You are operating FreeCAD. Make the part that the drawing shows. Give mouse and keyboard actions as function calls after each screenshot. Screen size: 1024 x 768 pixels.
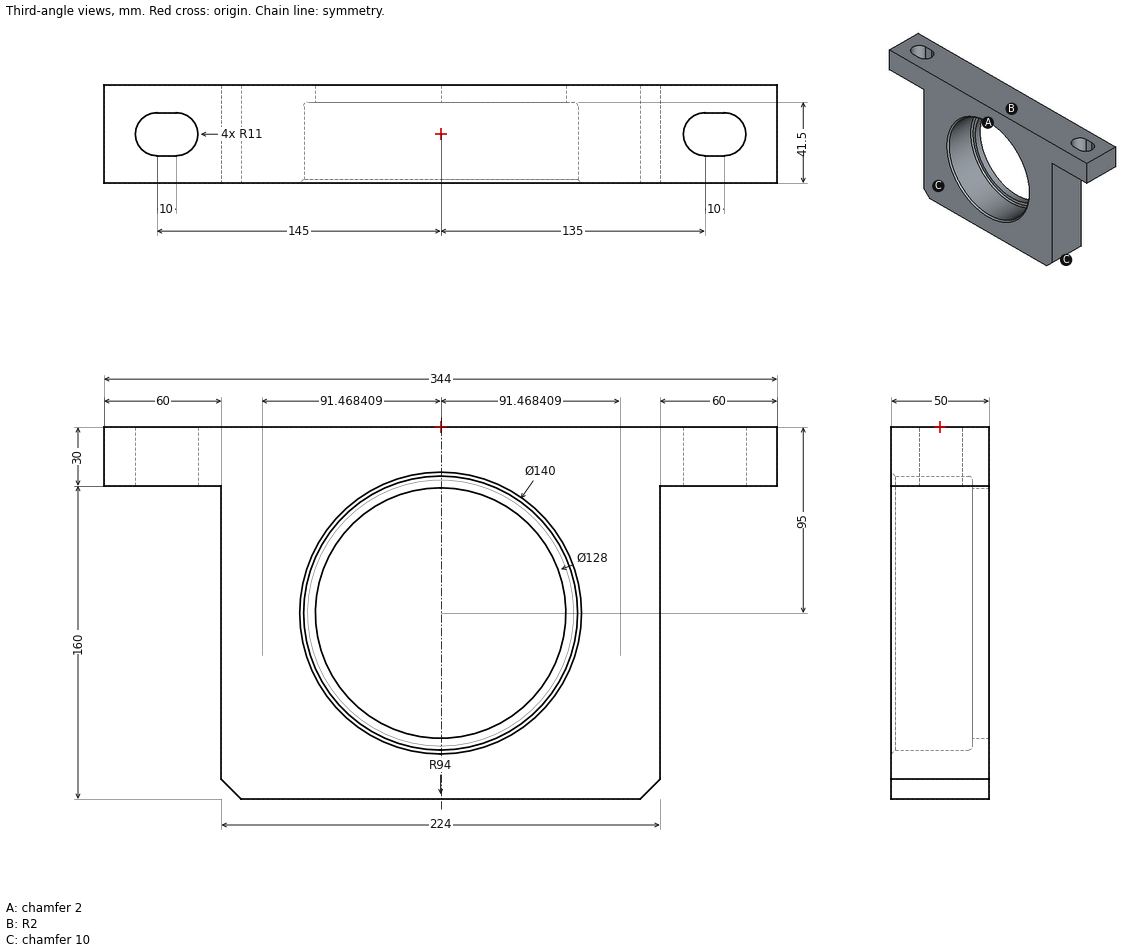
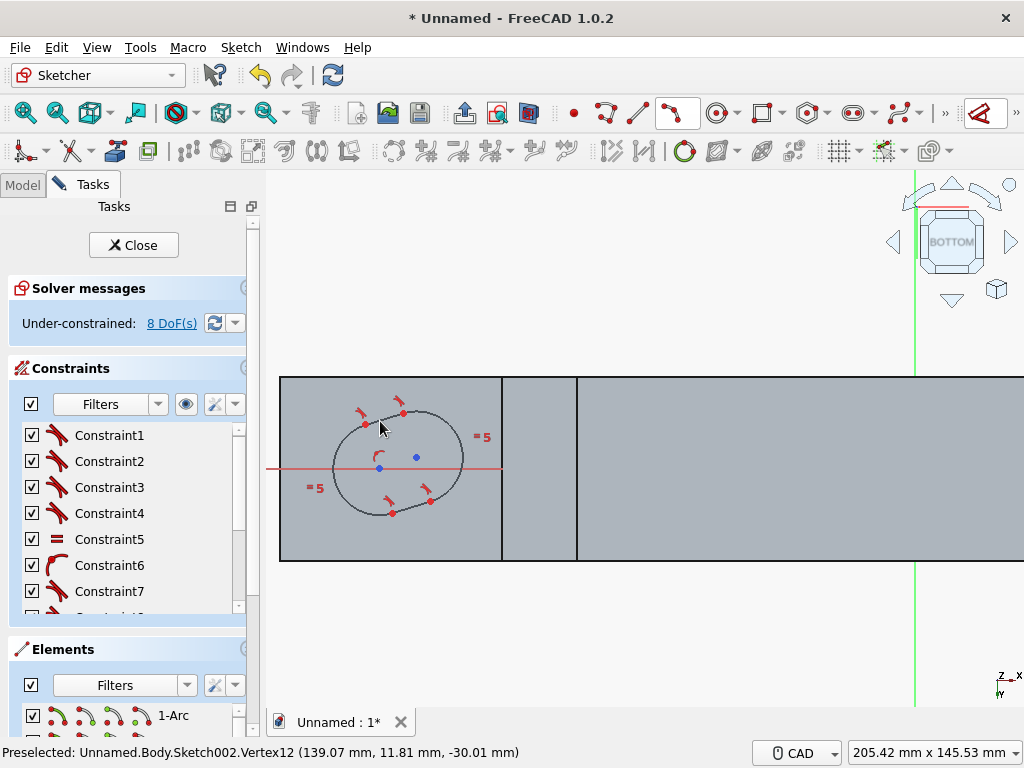
click(381, 420)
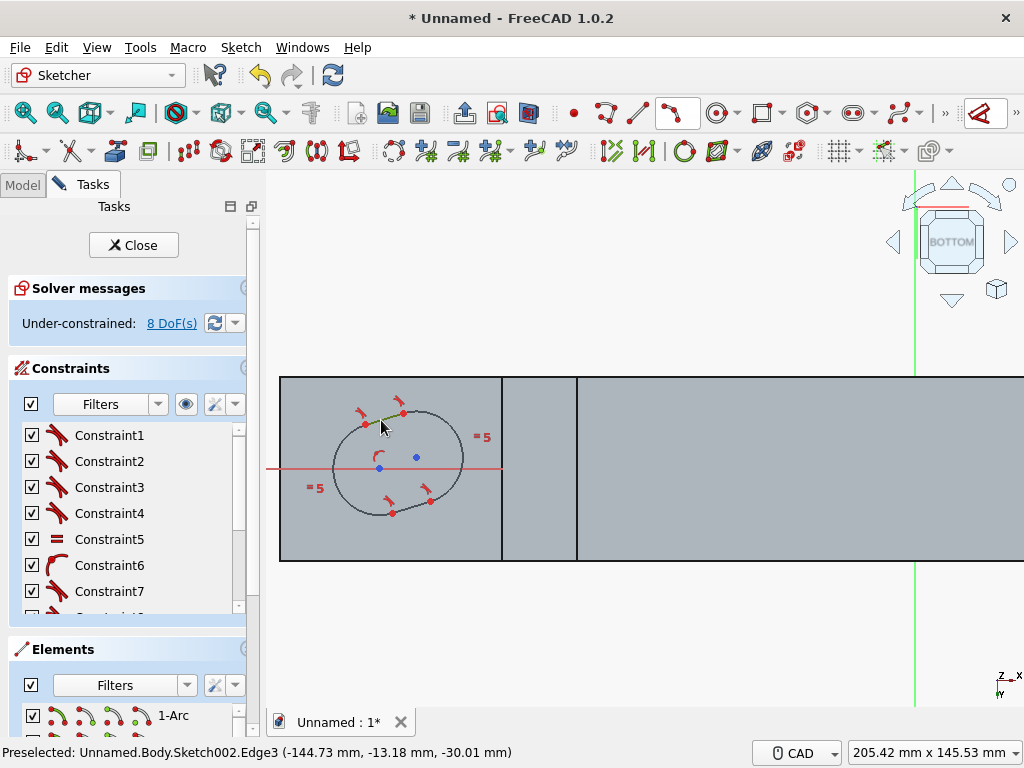
key(h)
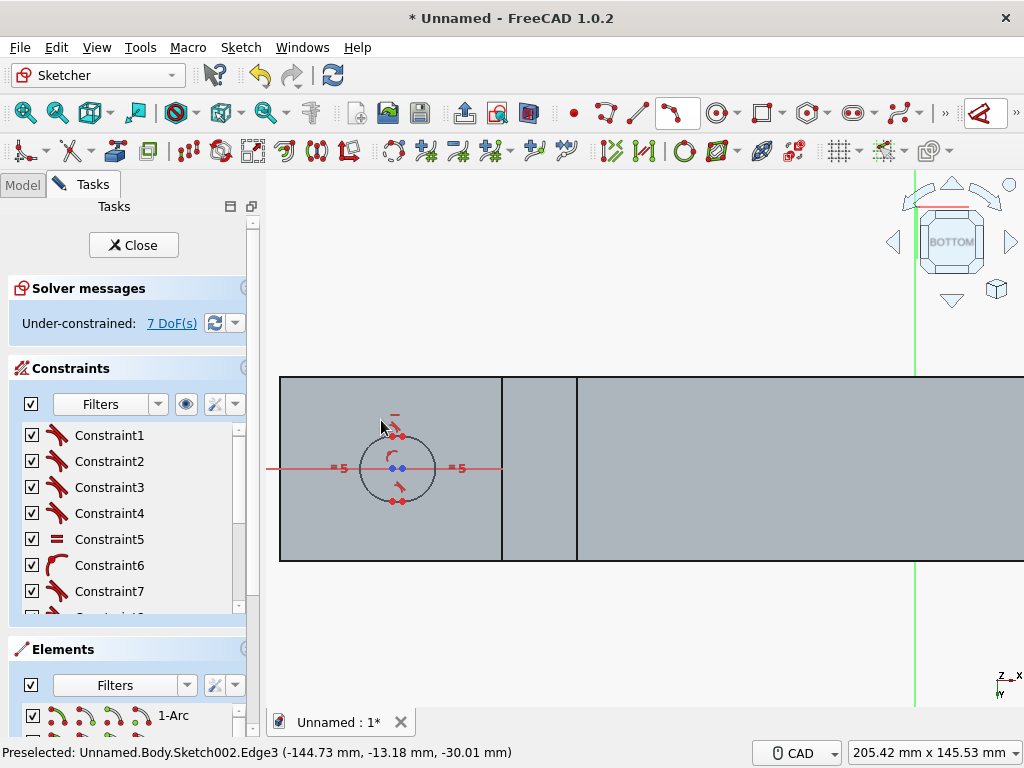
scroll(380, 421, down, 5)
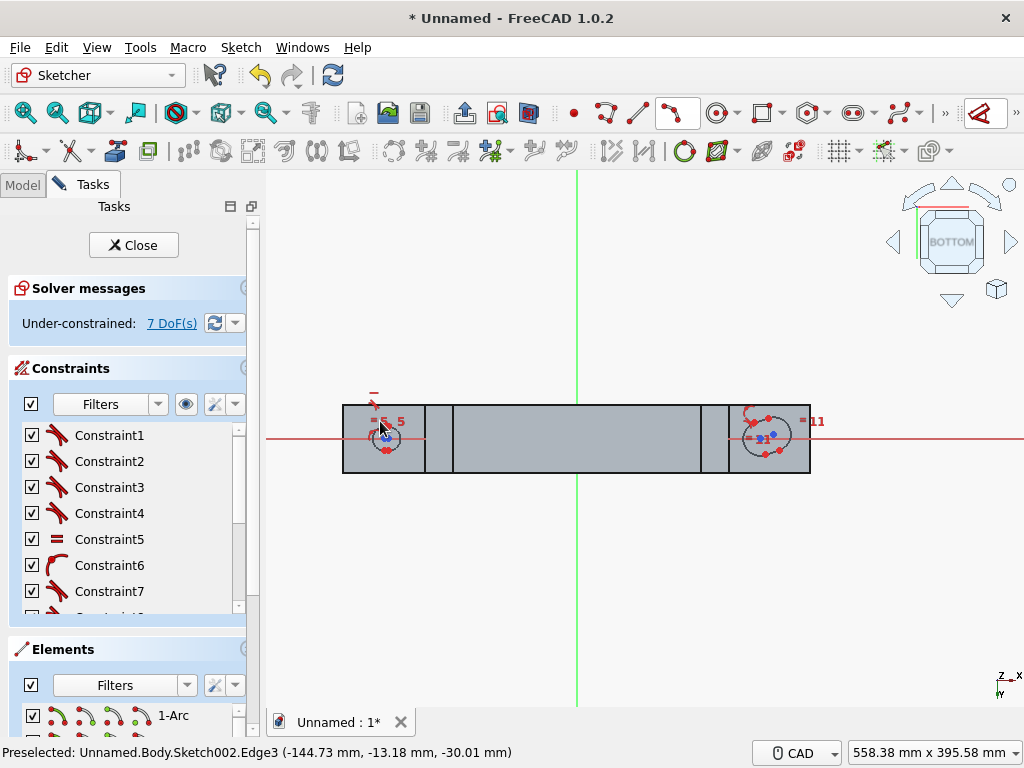
scroll(759, 422, up, 6)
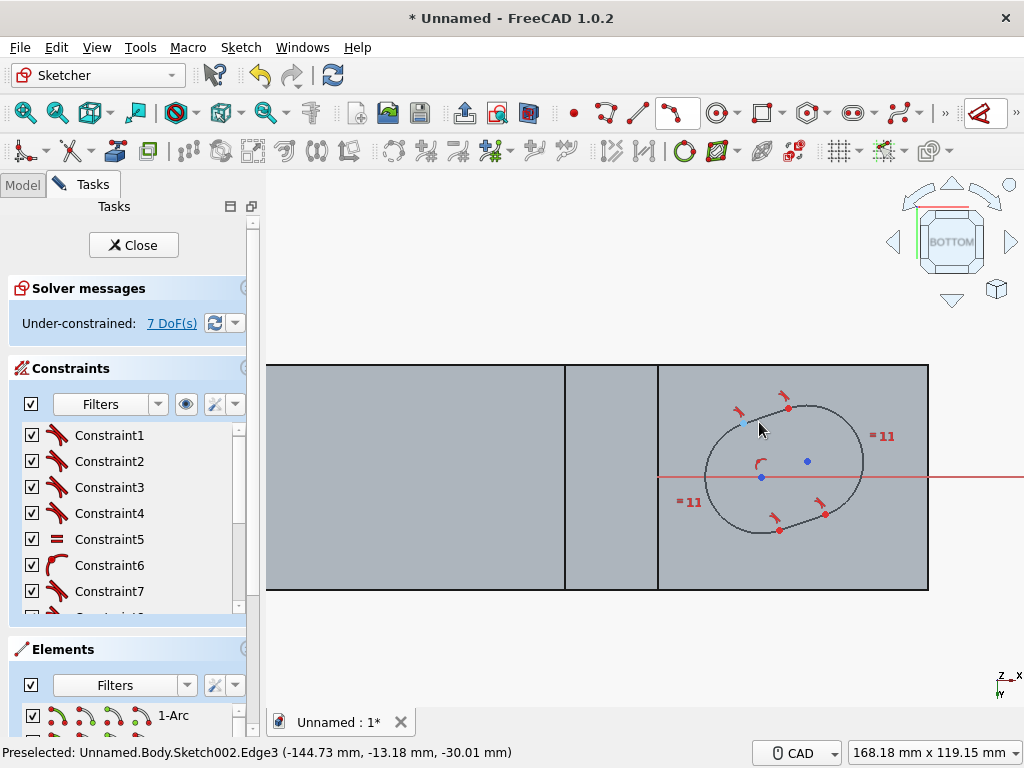
click(757, 419)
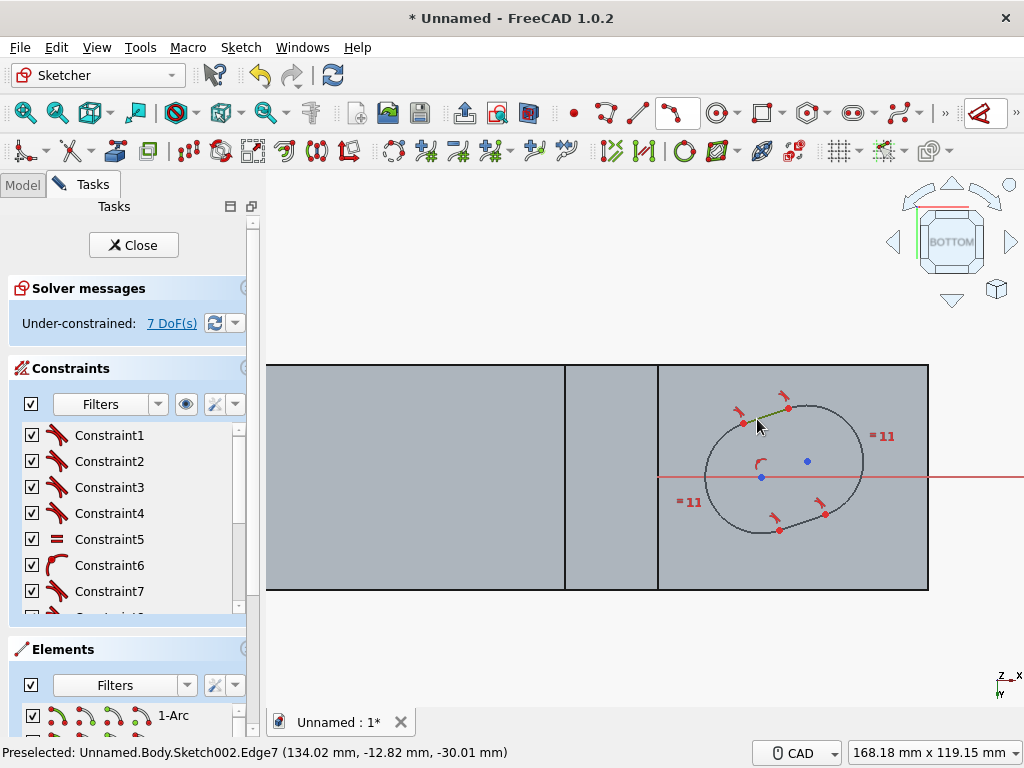
key(h)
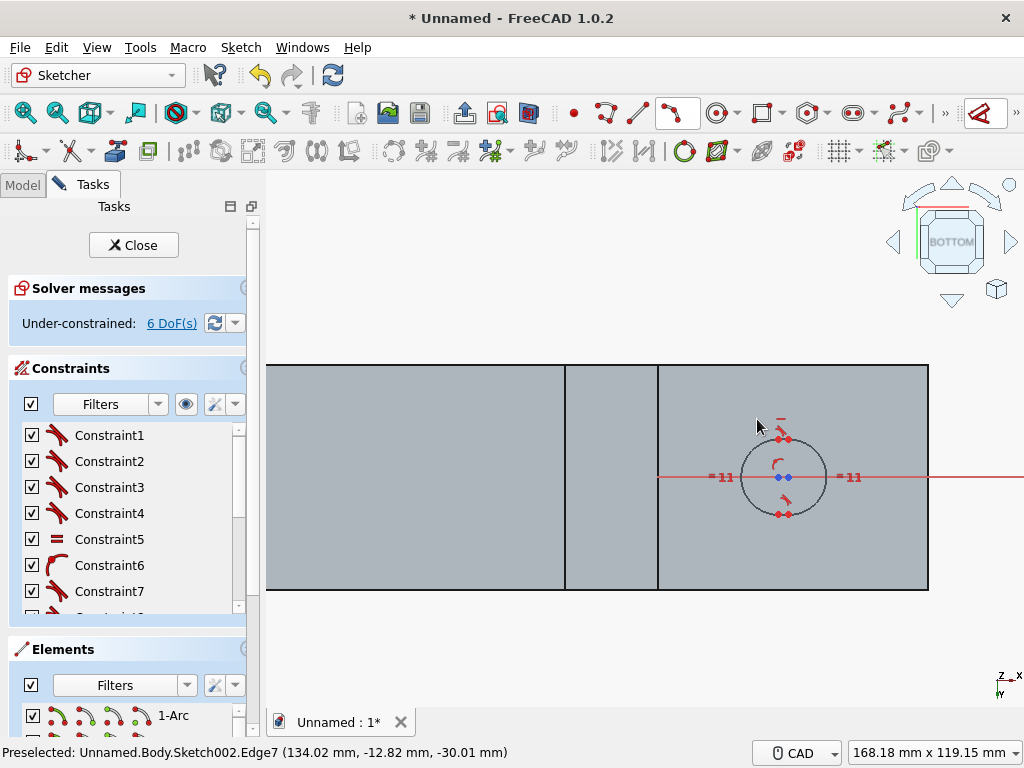
scroll(759, 422, down, 6)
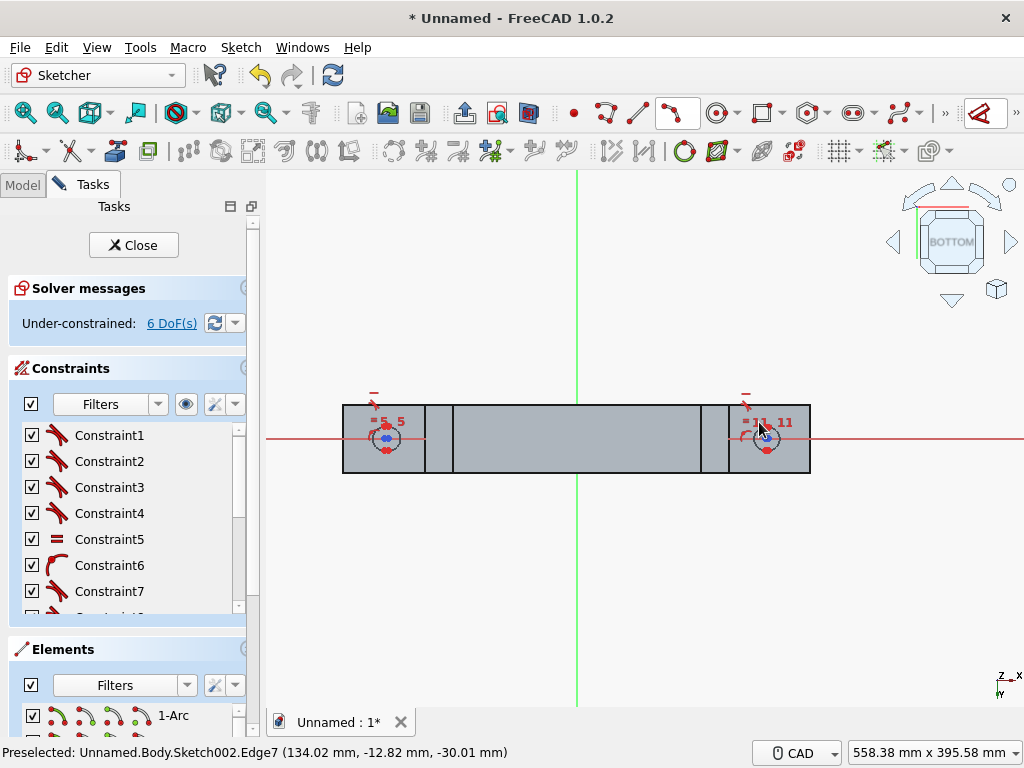
scroll(375, 432, up, 4)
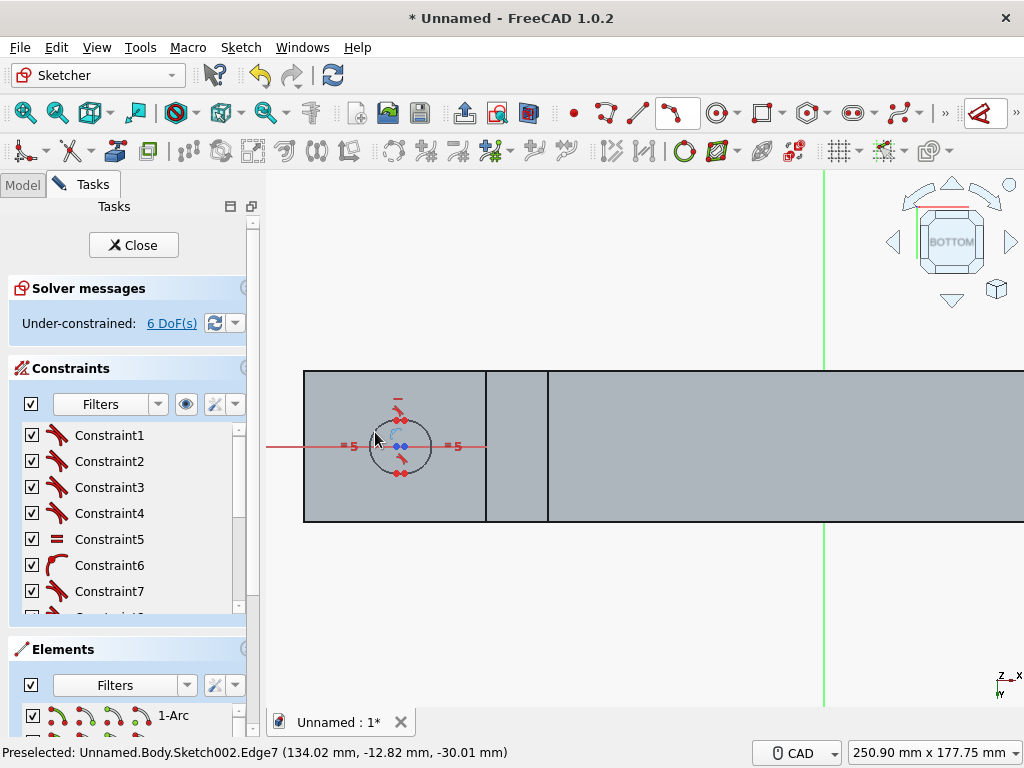
click(375, 431)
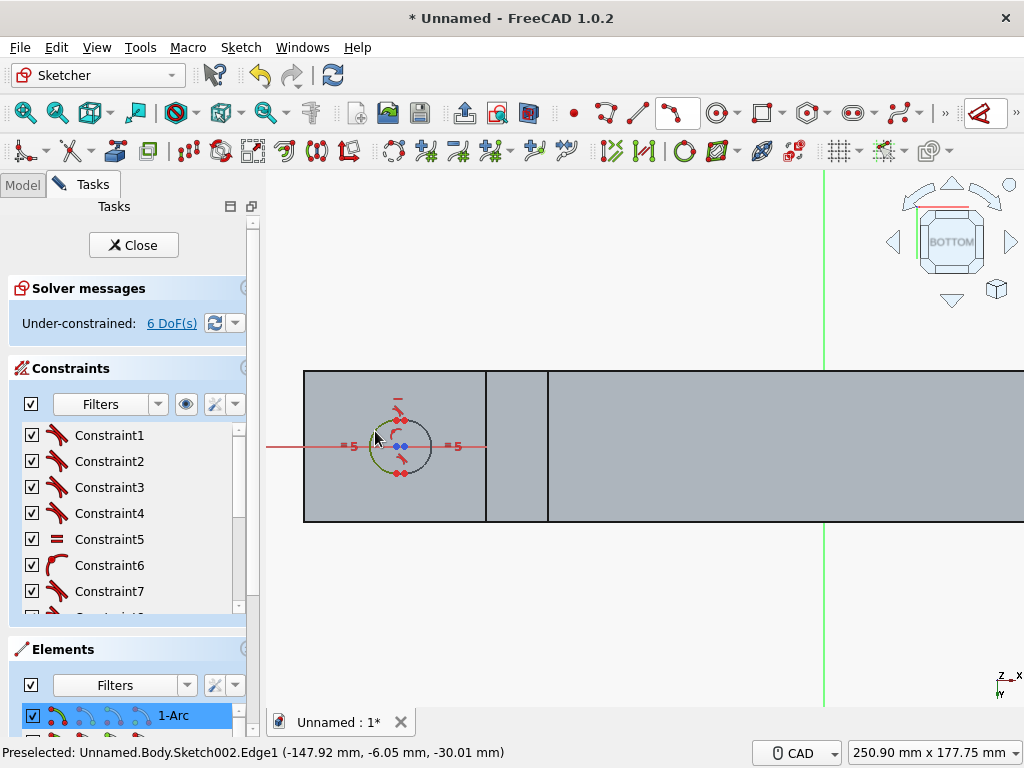
scroll(374, 432, down, 4)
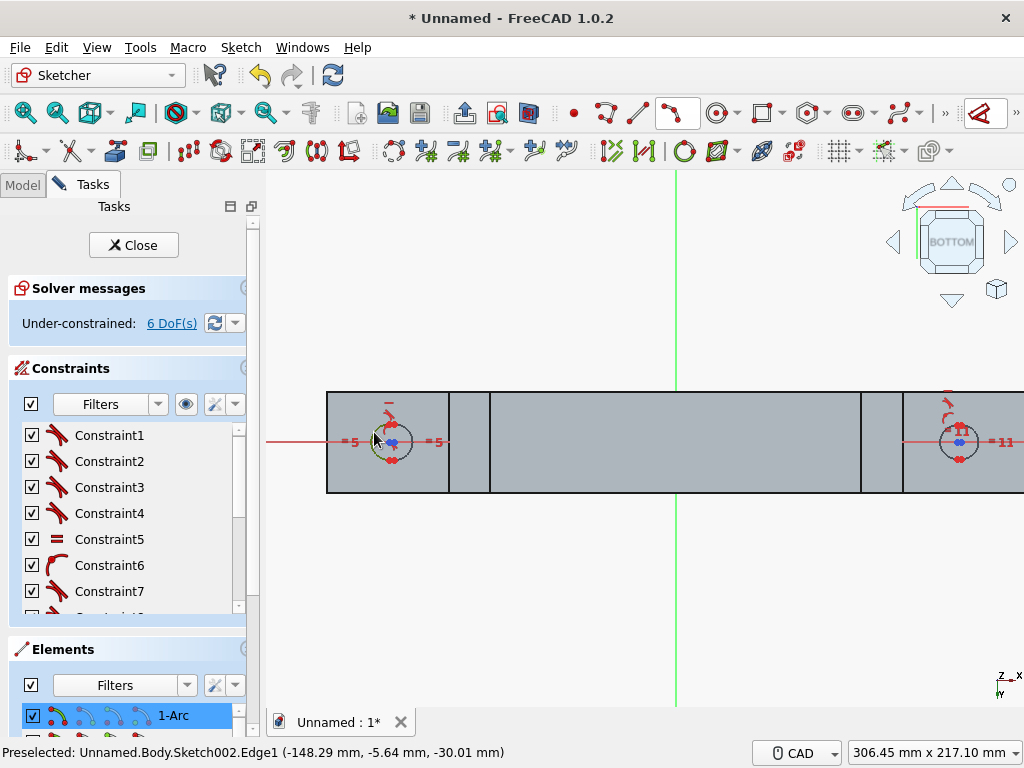
scroll(756, 432, up, 4)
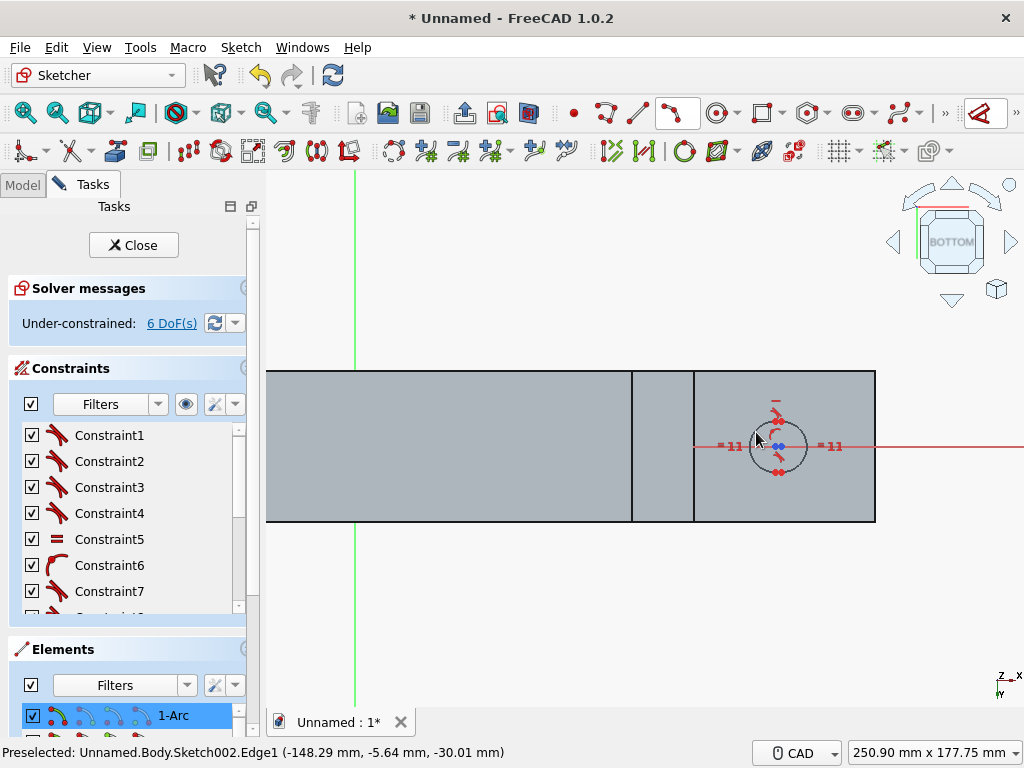
click(755, 432)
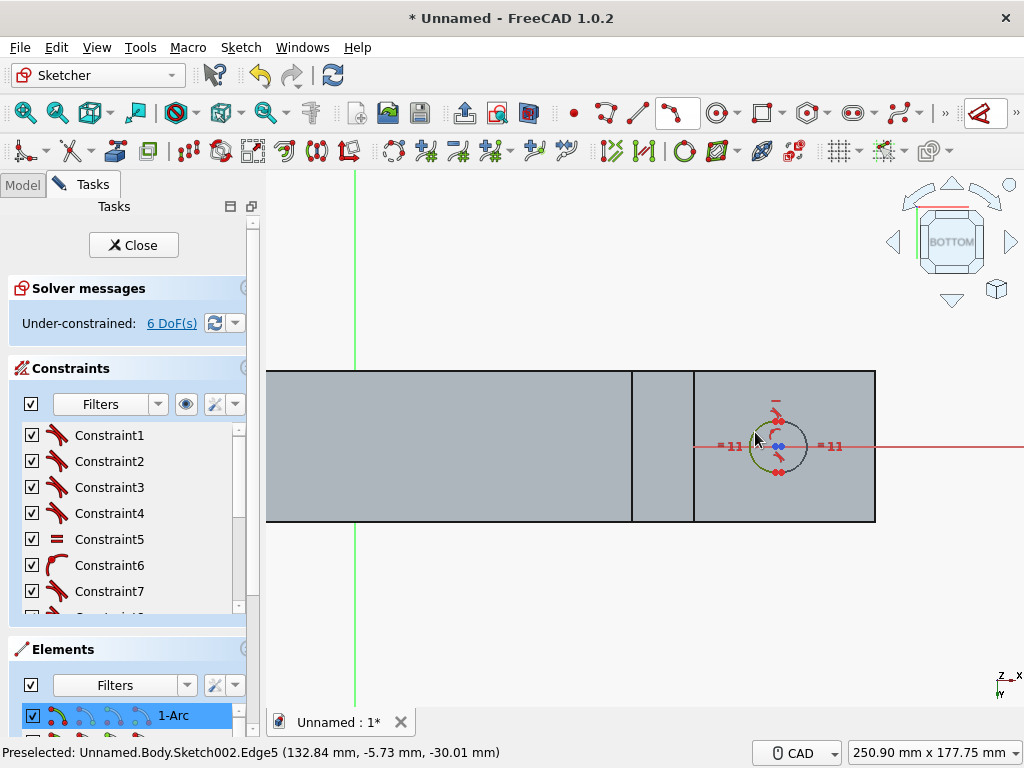
key(e)